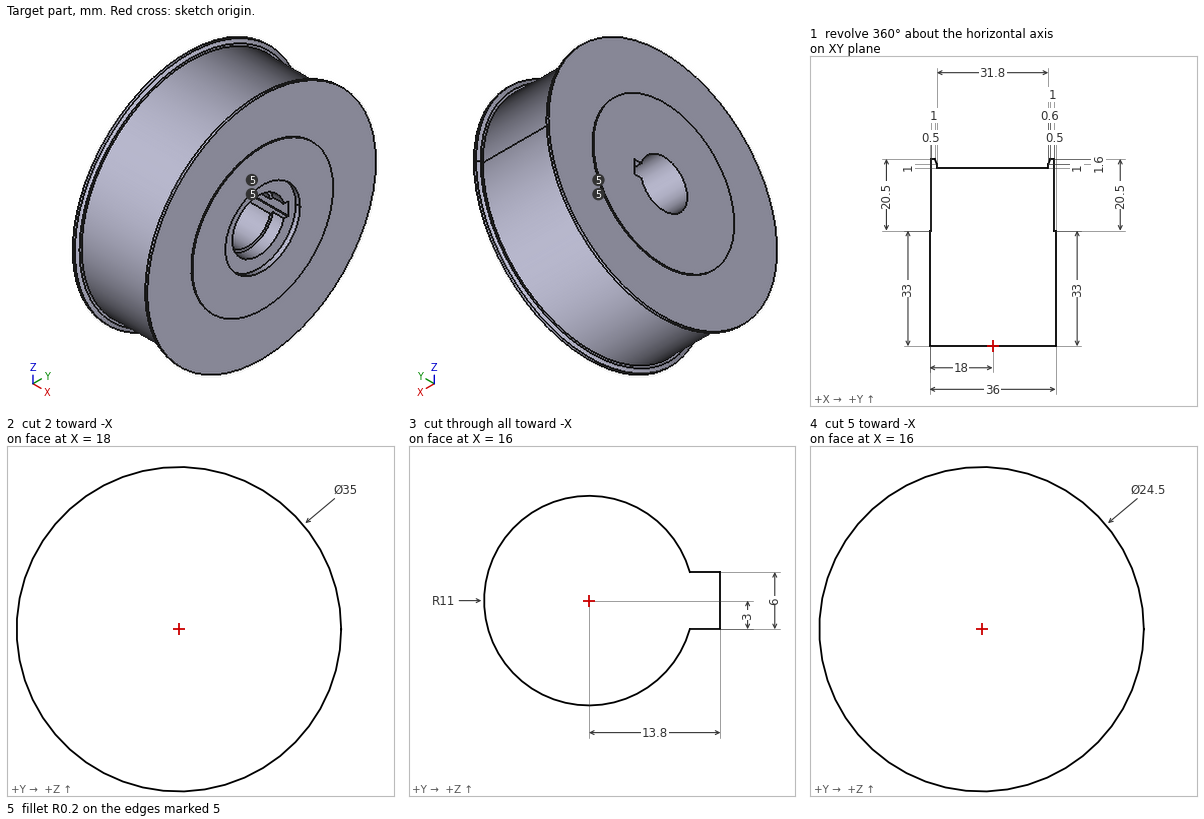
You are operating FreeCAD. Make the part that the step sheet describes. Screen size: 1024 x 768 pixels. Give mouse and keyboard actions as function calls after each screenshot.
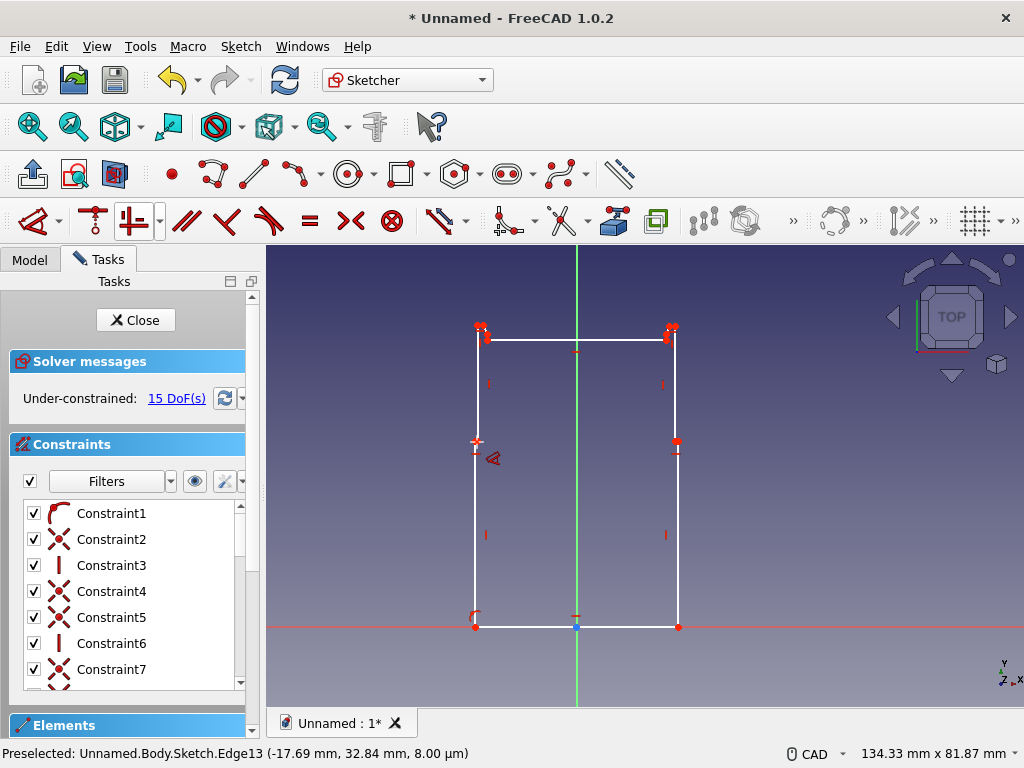
scroll(674, 326, up, 11)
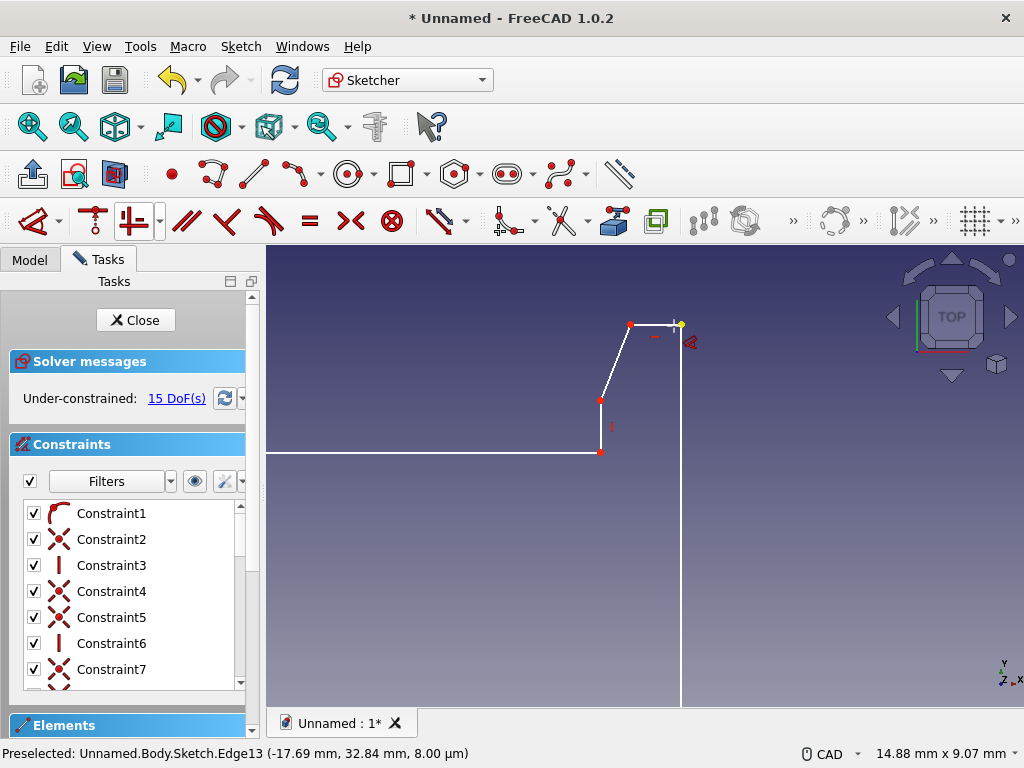
click(666, 325)
click(656, 291)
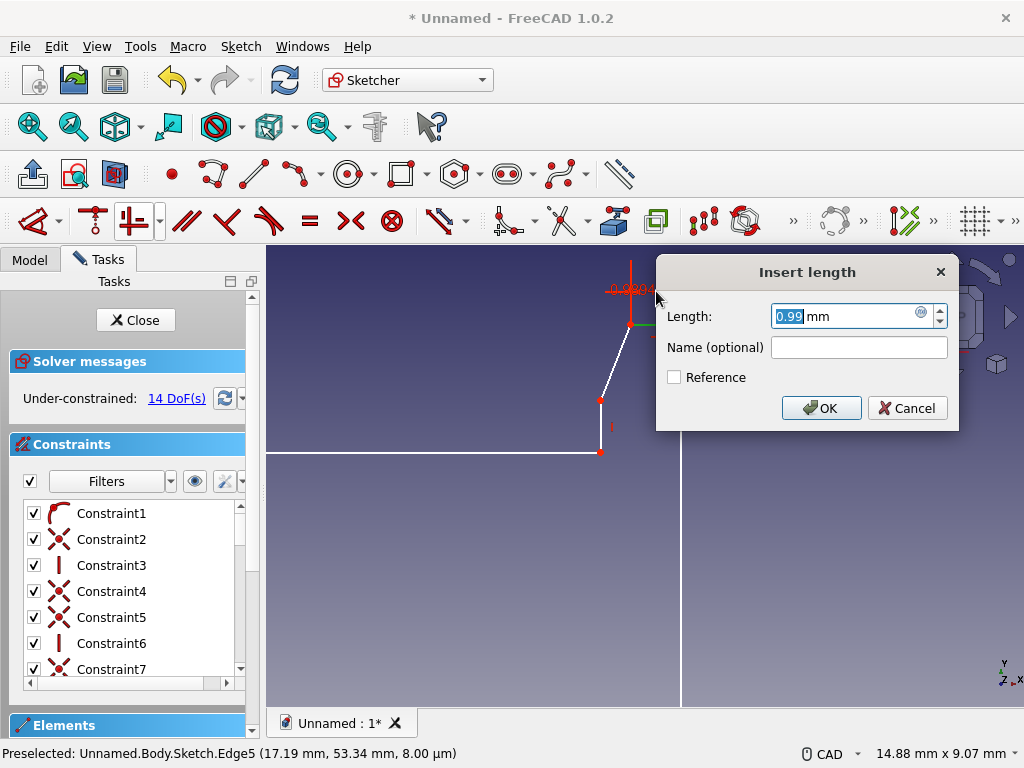
text(1)
key(Return)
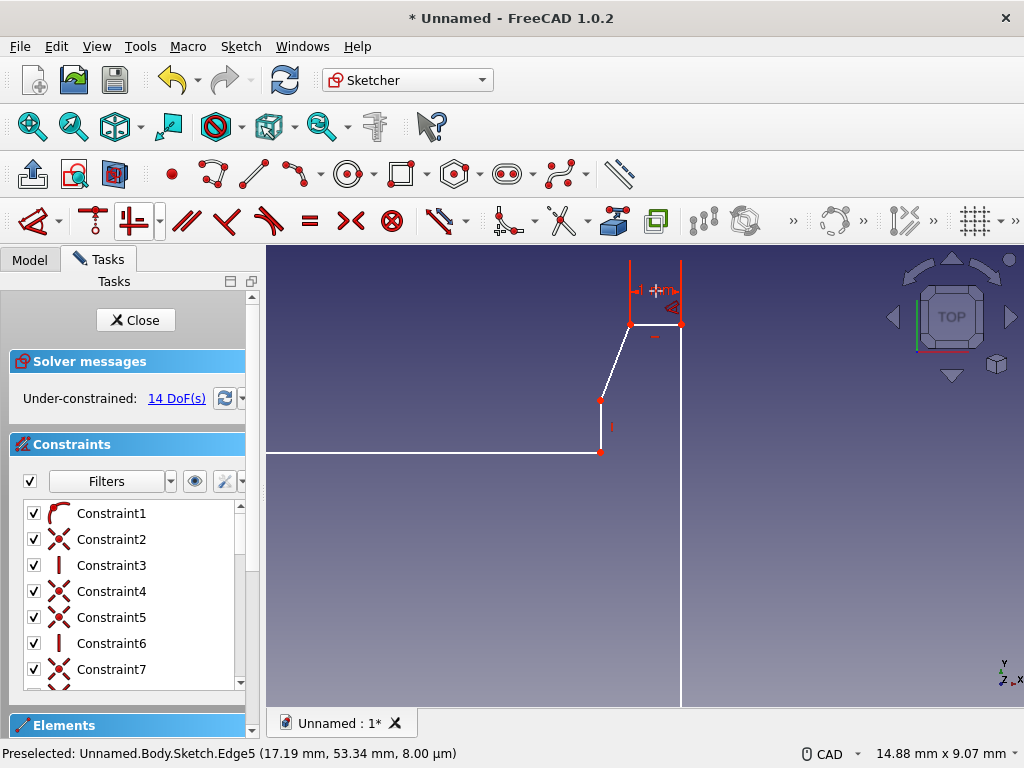
click(601, 416)
click(635, 427)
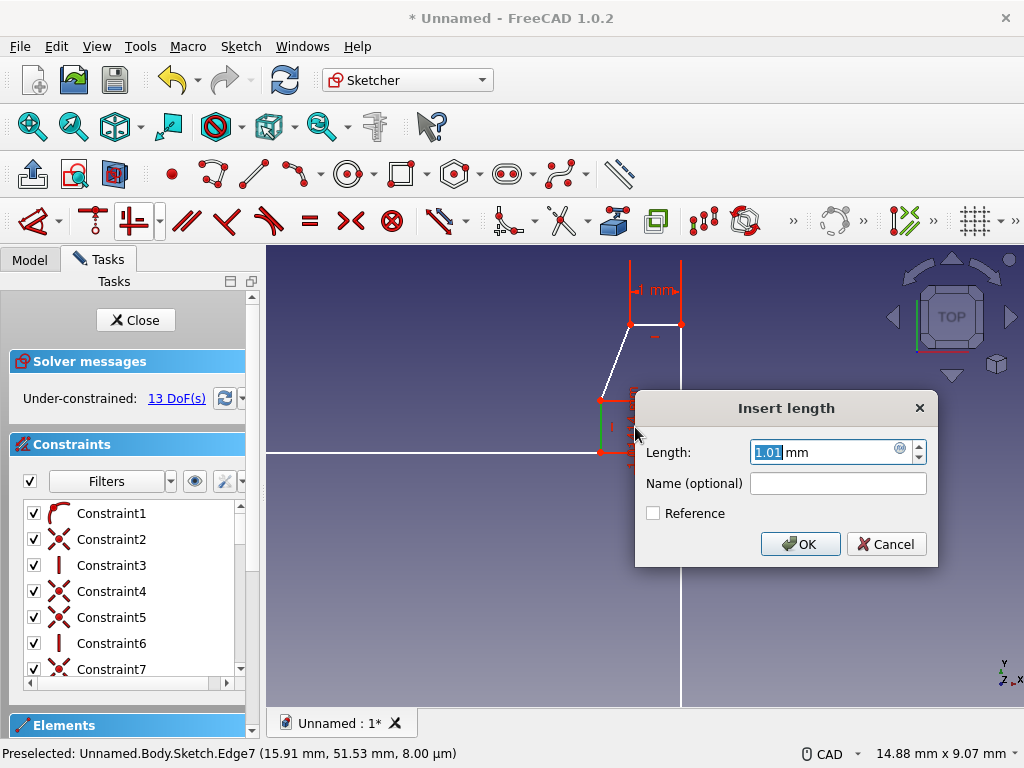
text(1)
key(Return)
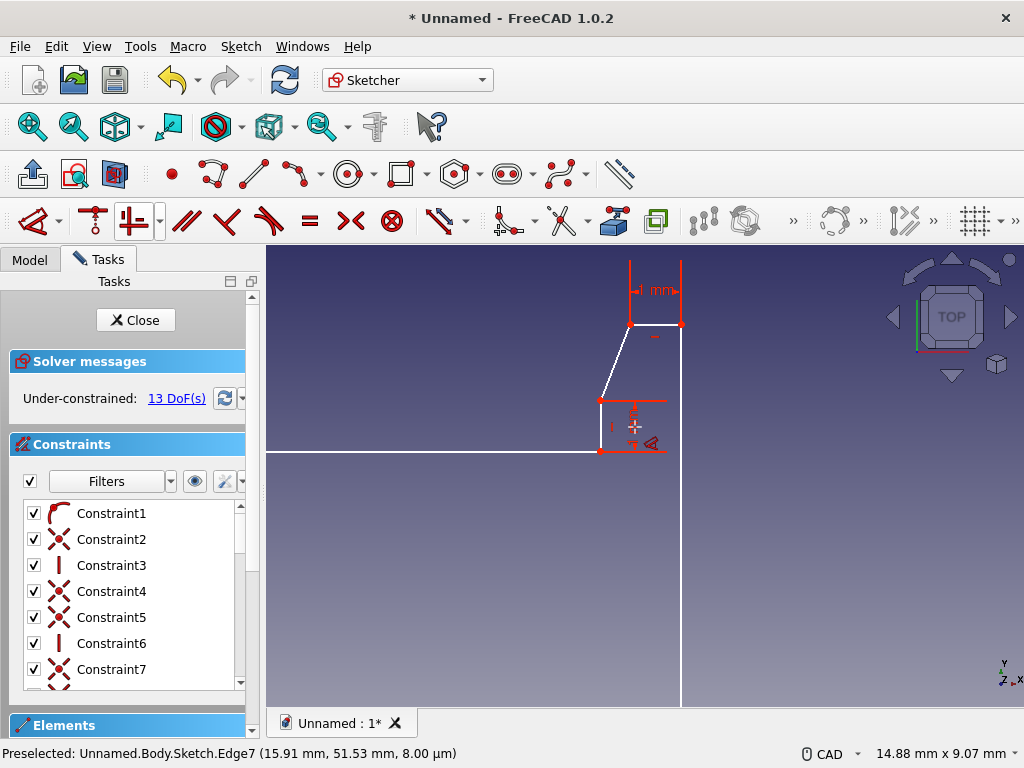
scroll(674, 326, down, 11)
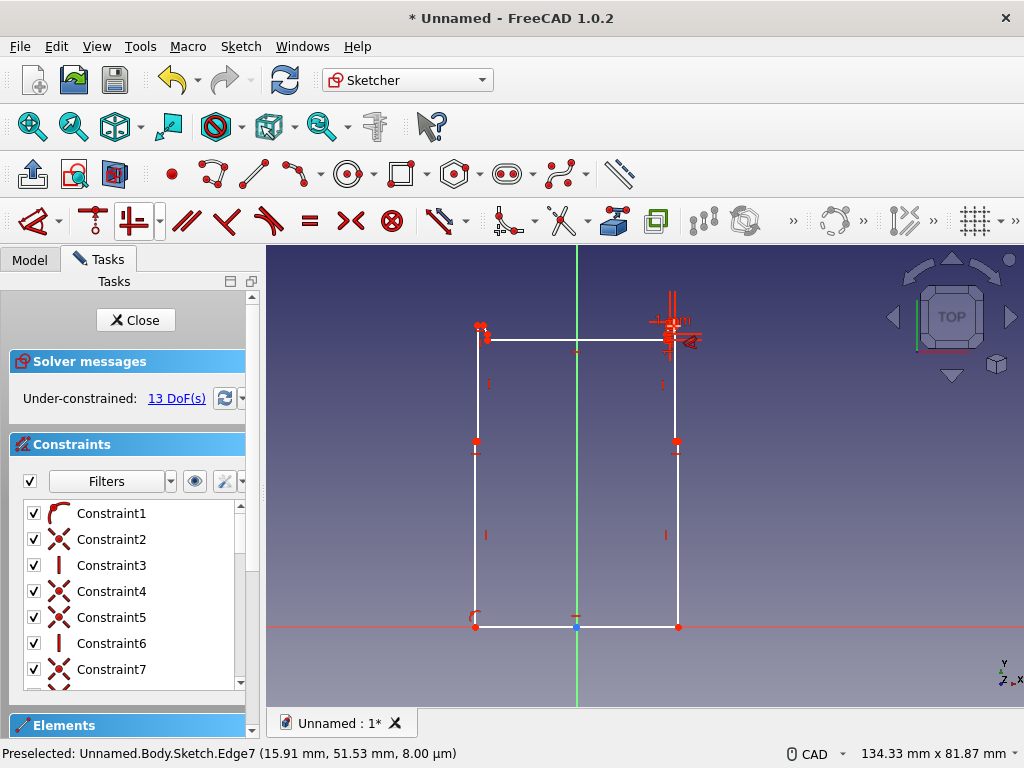
scroll(487, 338, up, 11)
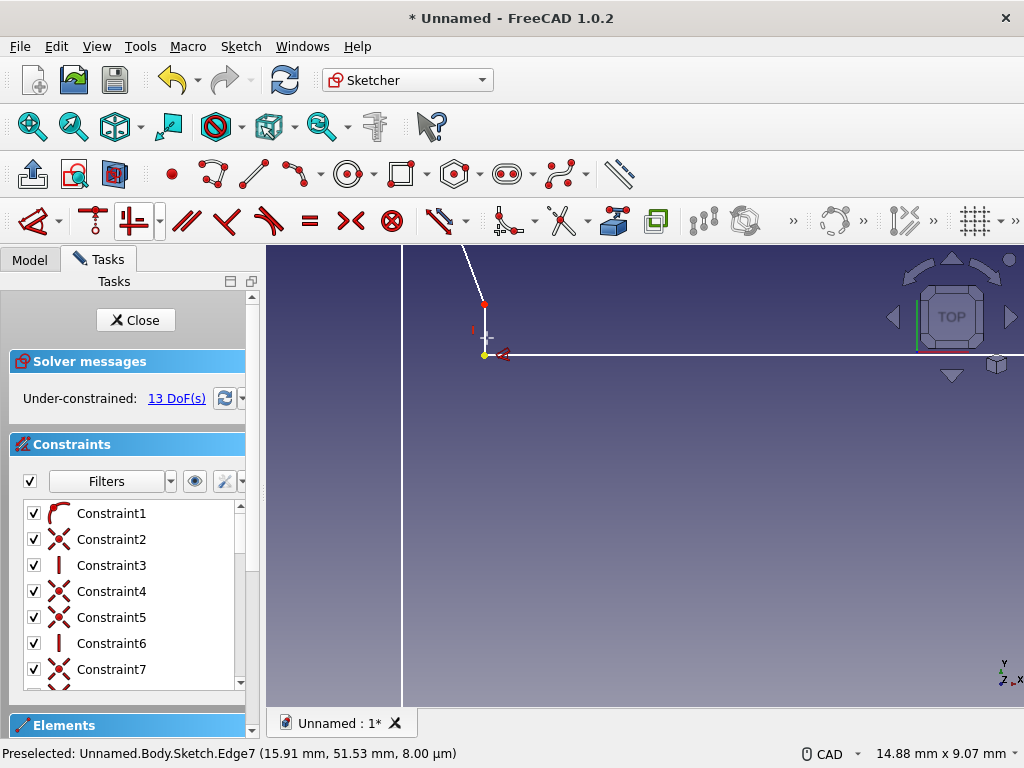
click(485, 340)
click(451, 330)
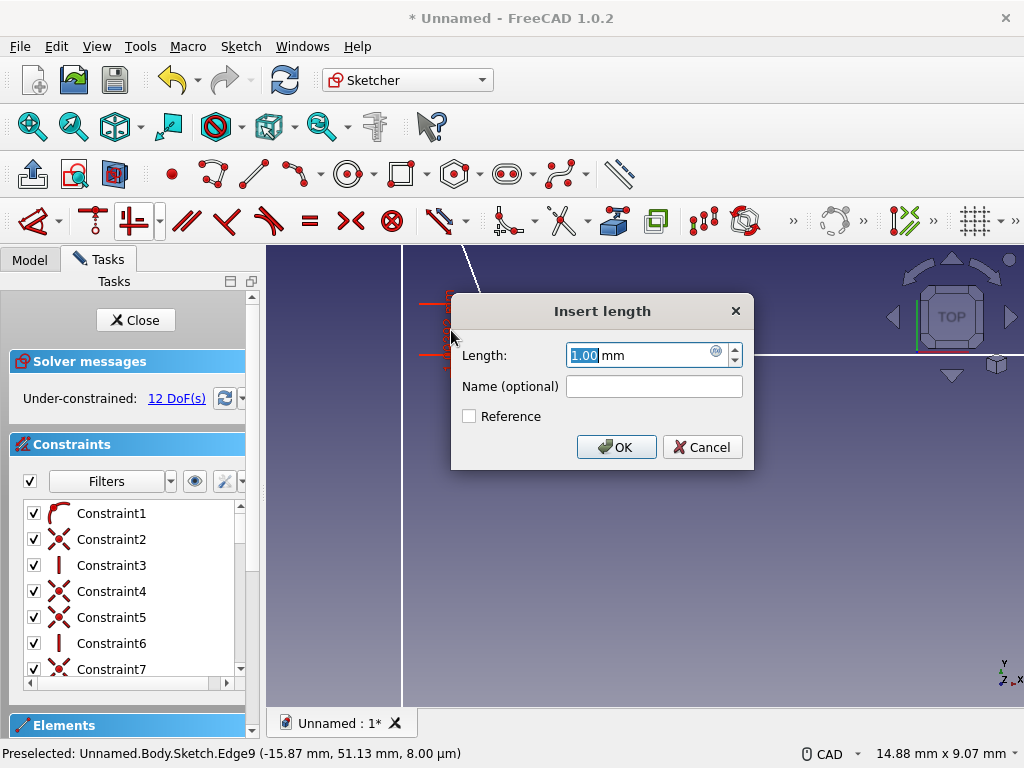
text(1)
key(Return)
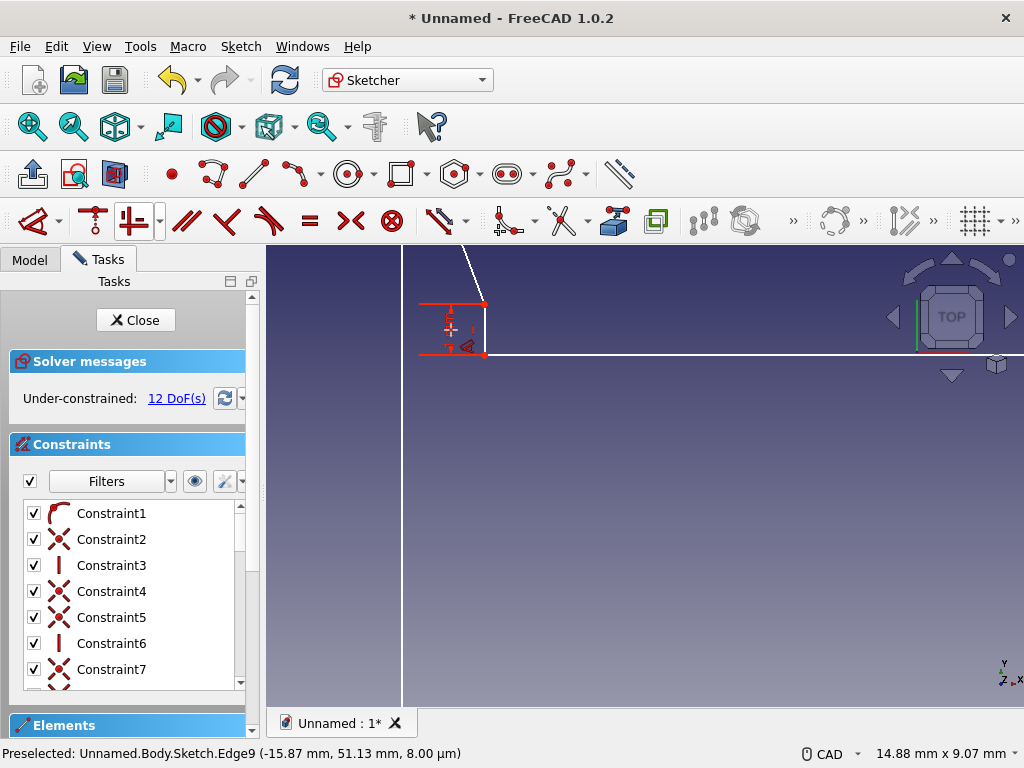
scroll(487, 338, down, 11)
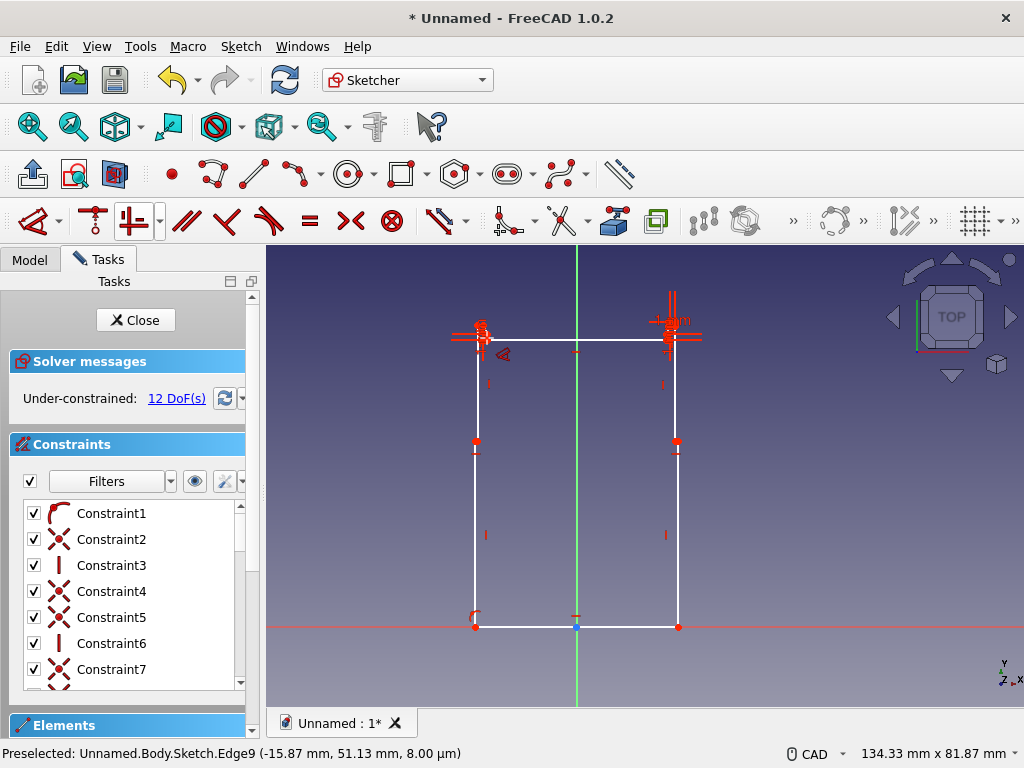
scroll(482, 325, up, 11)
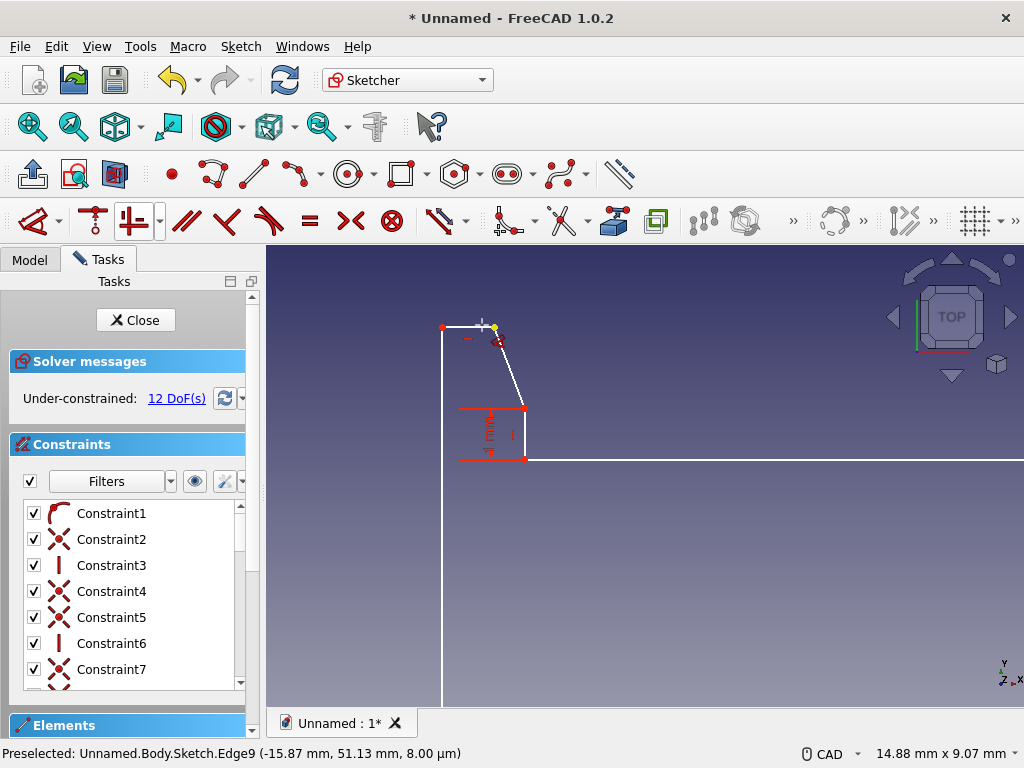
click(479, 327)
click(468, 293)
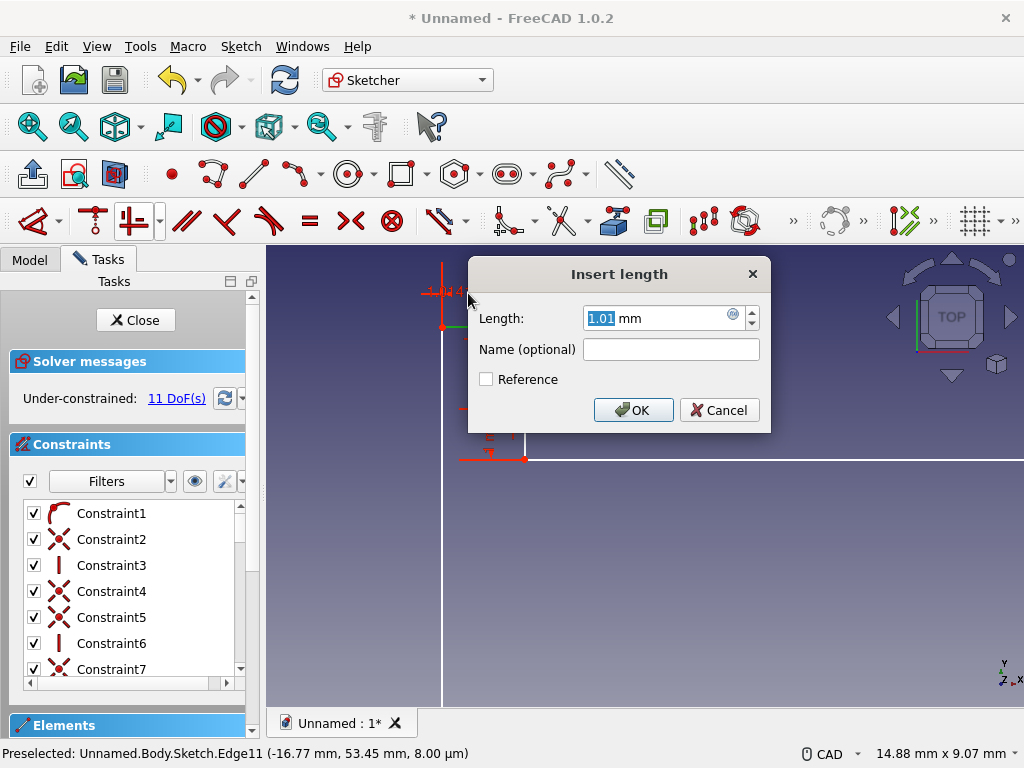
text(1)
key(Return)